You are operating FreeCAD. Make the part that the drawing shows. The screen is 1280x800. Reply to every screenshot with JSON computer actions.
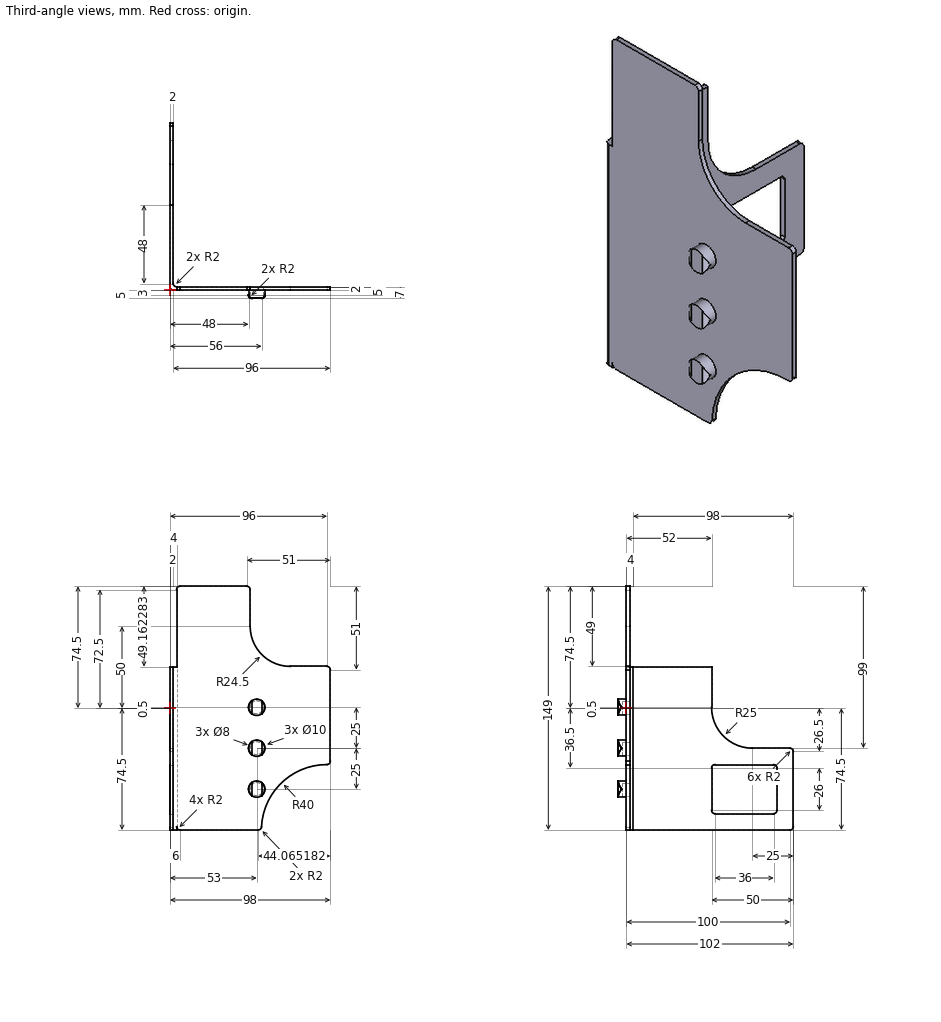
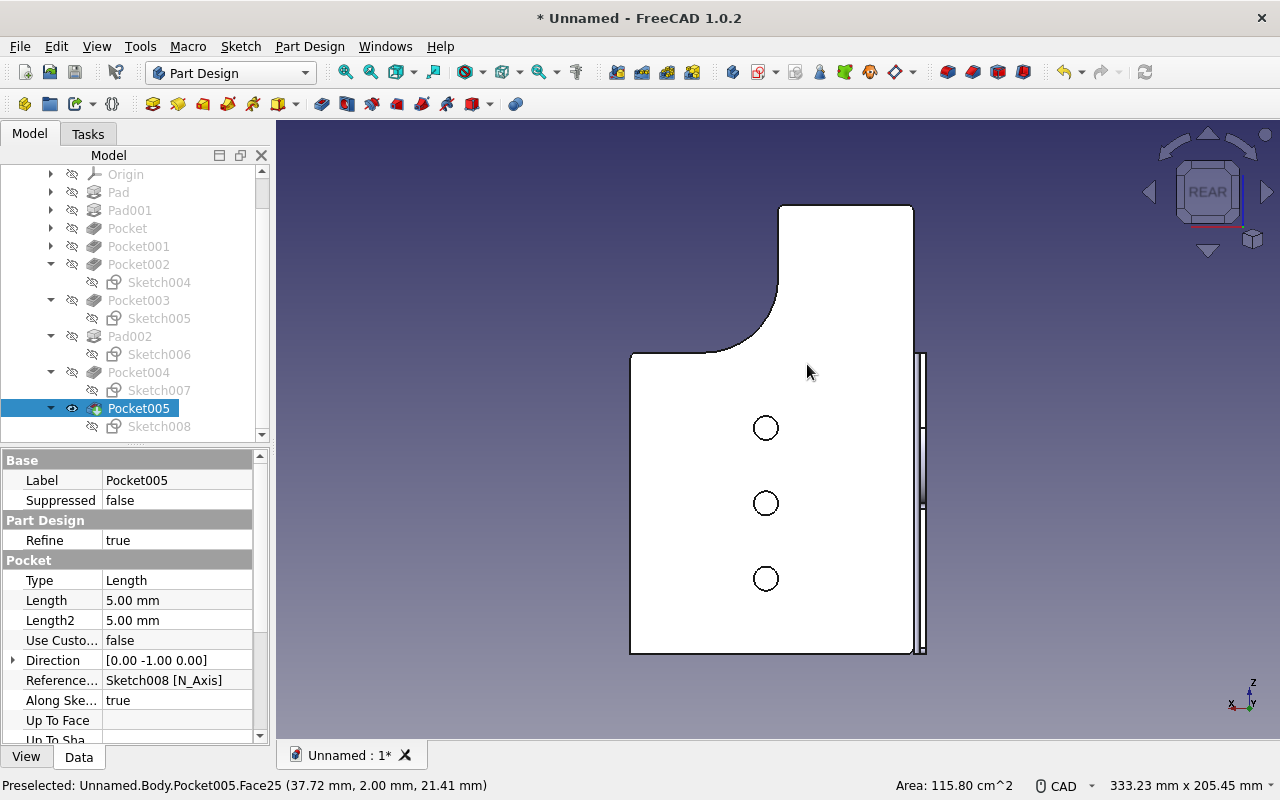
{"action": "left_click", "coordinate": [758, 72]}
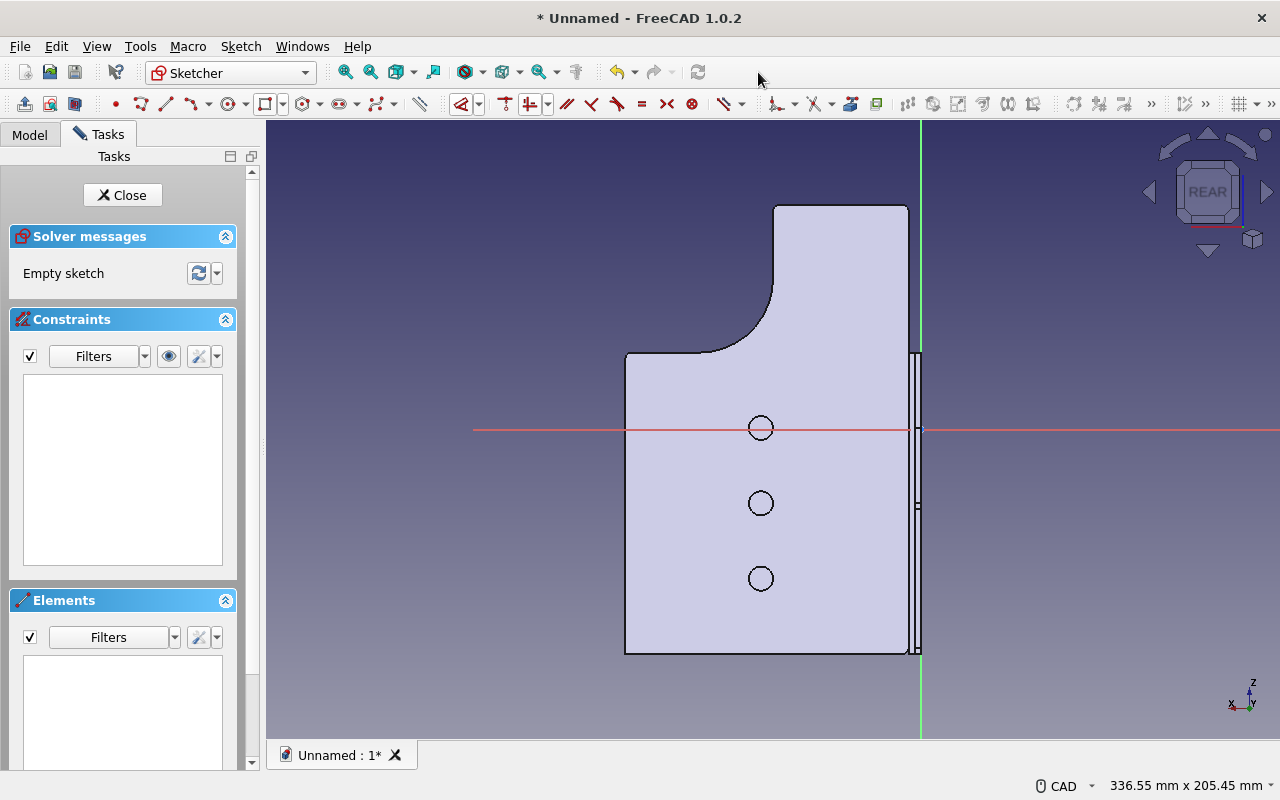
{"action": "scroll", "coordinate": [856, 678], "scroll_direction": "up", "scroll_amount": 3}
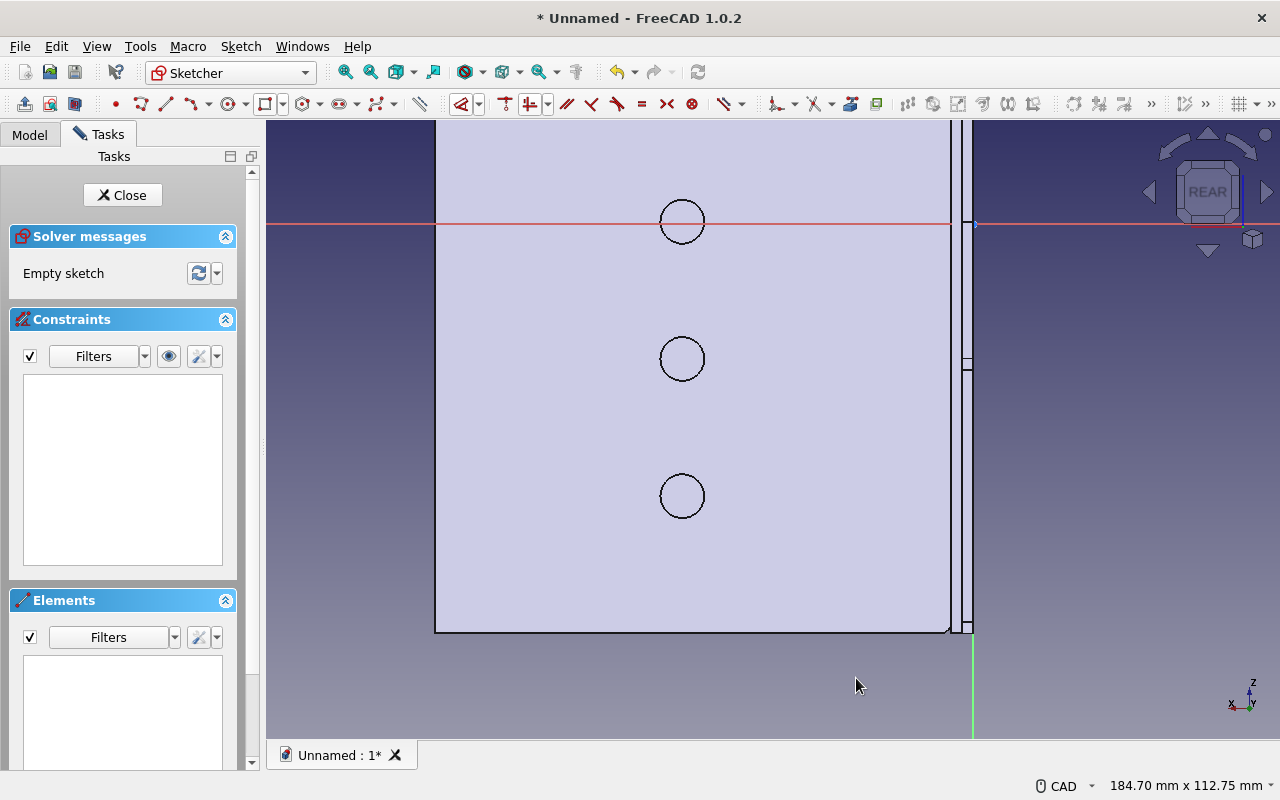
{"action": "key", "text": "g m"}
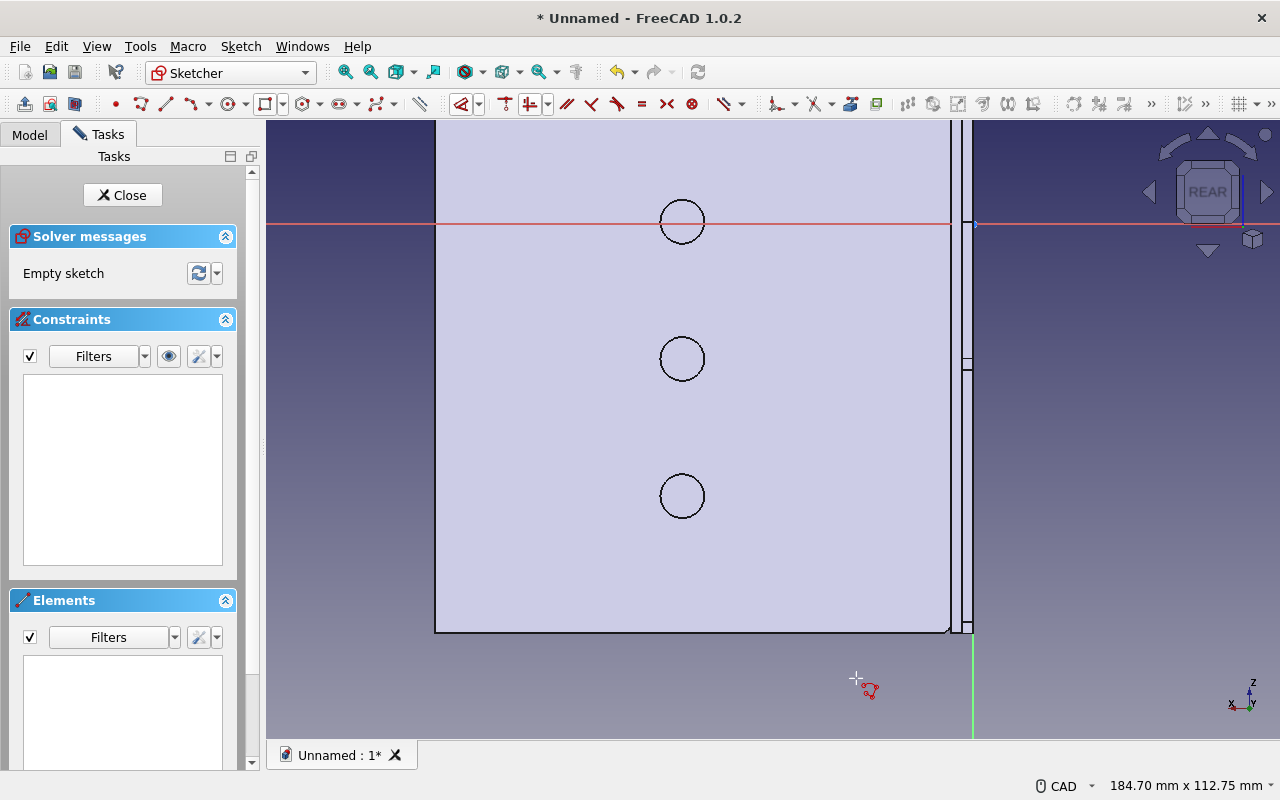
{"action": "left_click", "coordinate": [435, 403]}
{"action": "left_click", "coordinate": [435, 633]}
{"action": "left_click", "coordinate": [677, 633]}
{"action": "right_click", "coordinate": [677, 633]}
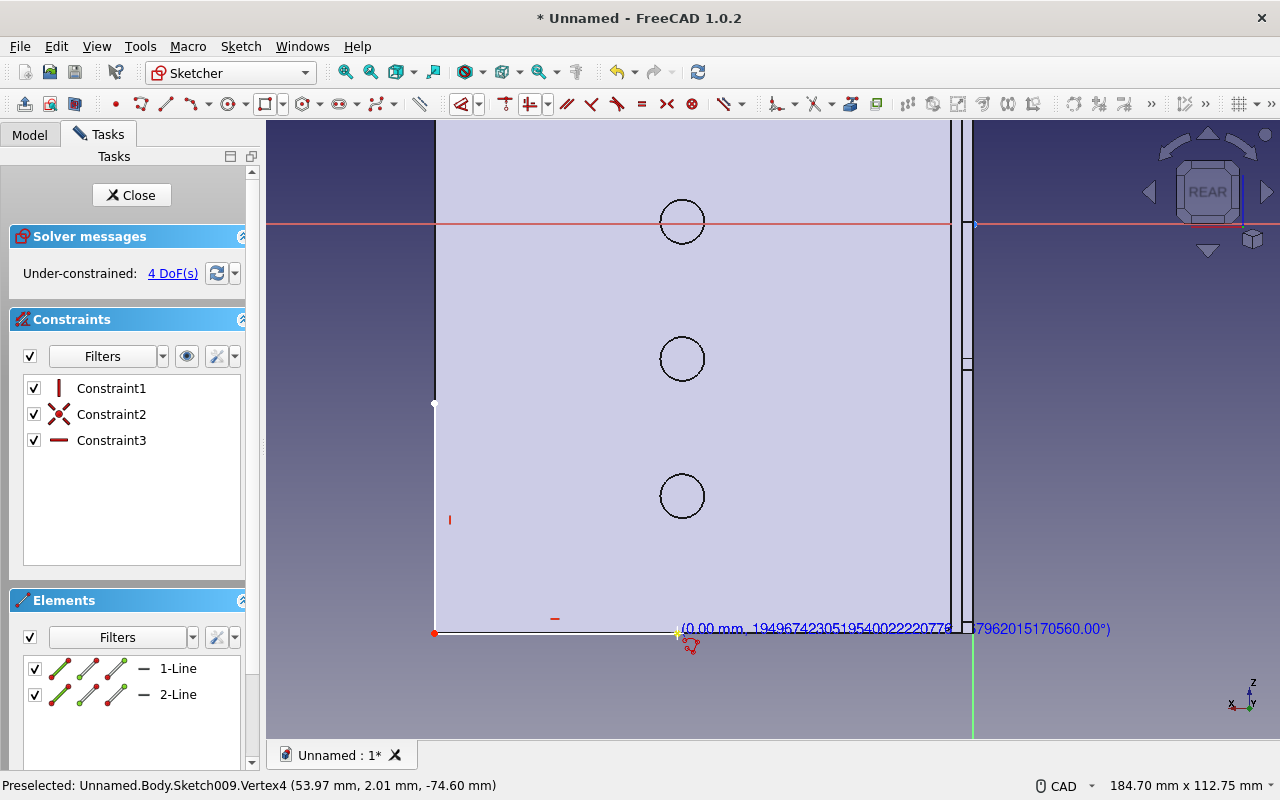
{"action": "key", "text": "g 3 a"}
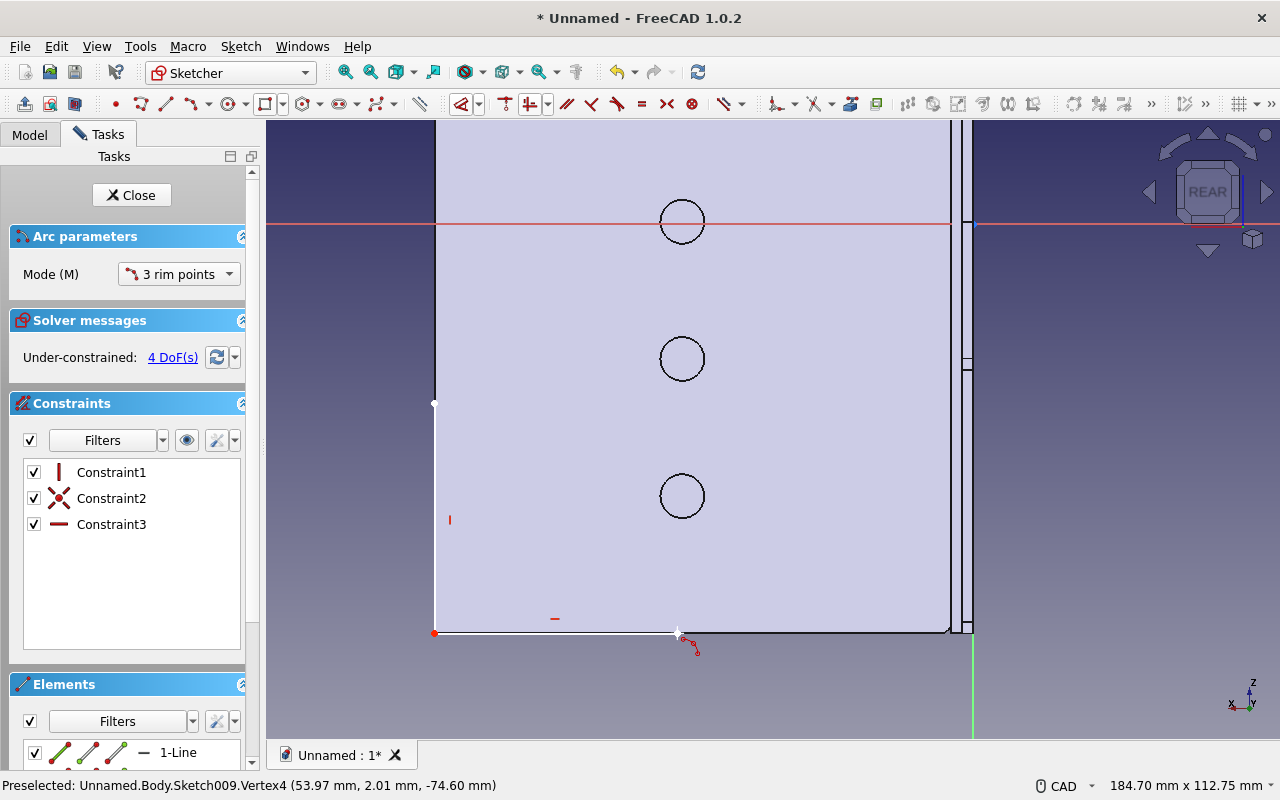
{"action": "left_click", "coordinate": [677, 634]}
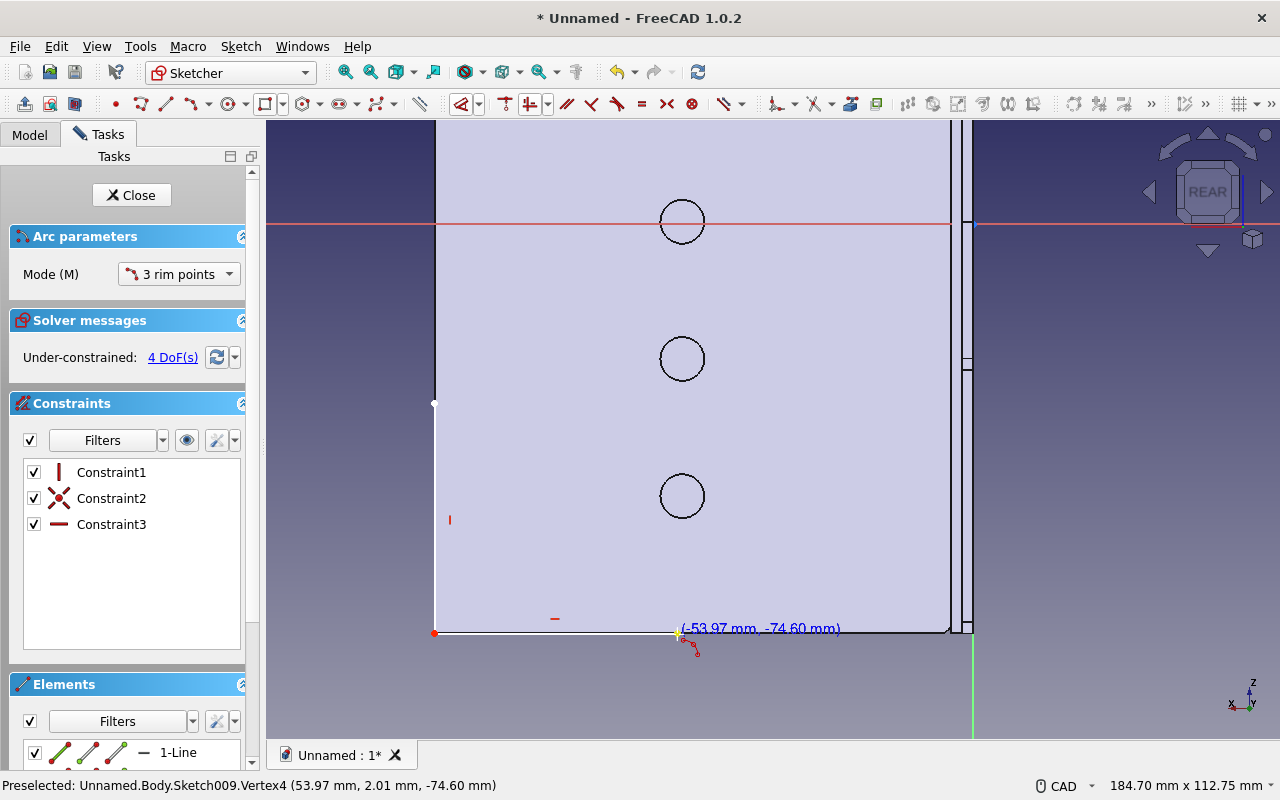
{"action": "scroll", "coordinate": [666, 623], "scroll_direction": "up", "scroll_amount": 3}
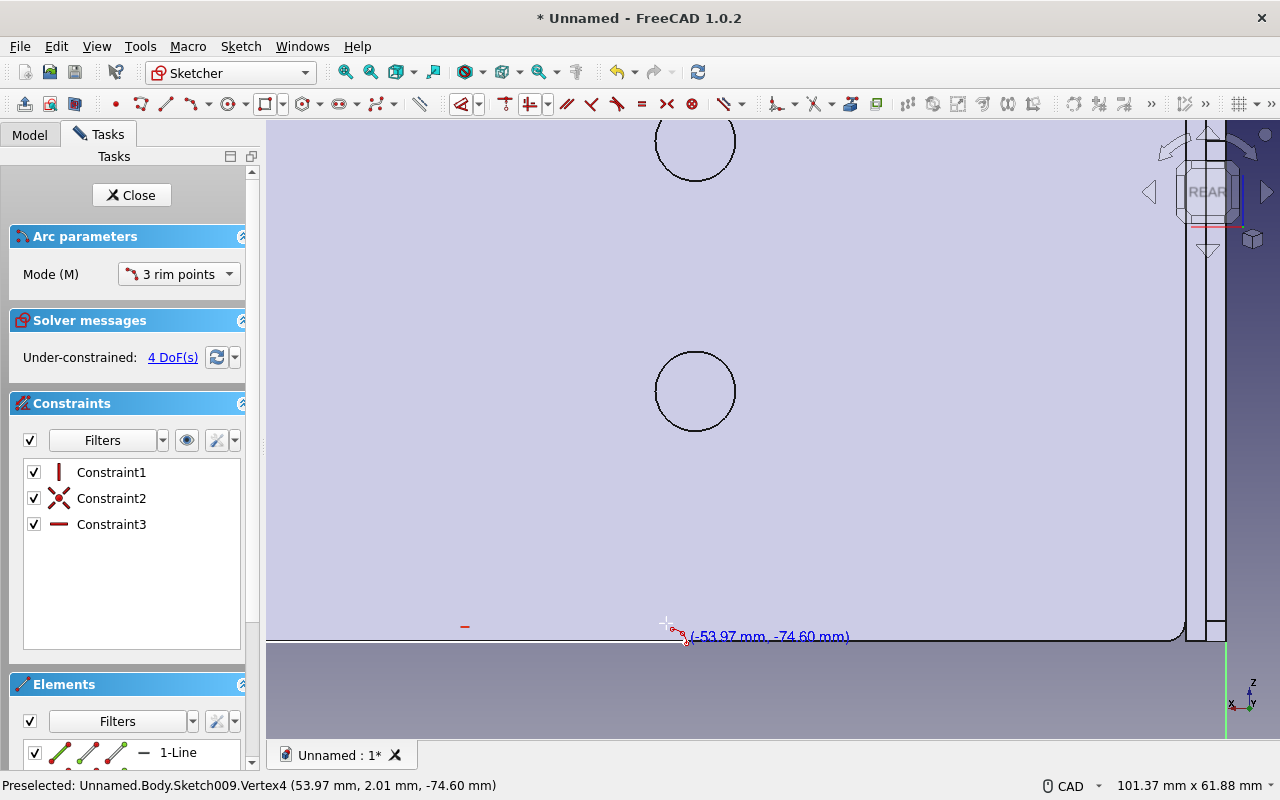
{"action": "left_click", "coordinate": [666, 622]}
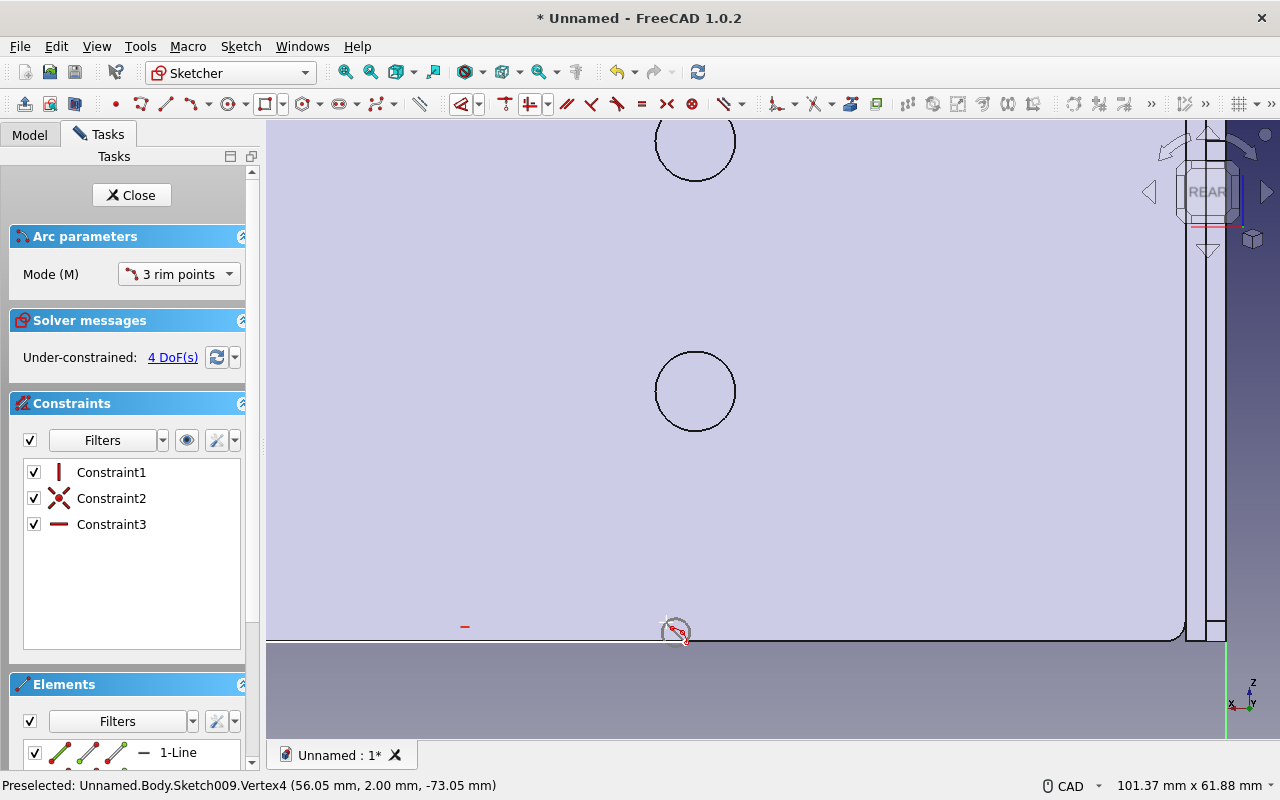
{"action": "scroll", "coordinate": [672, 636], "scroll_direction": "up", "scroll_amount": 6}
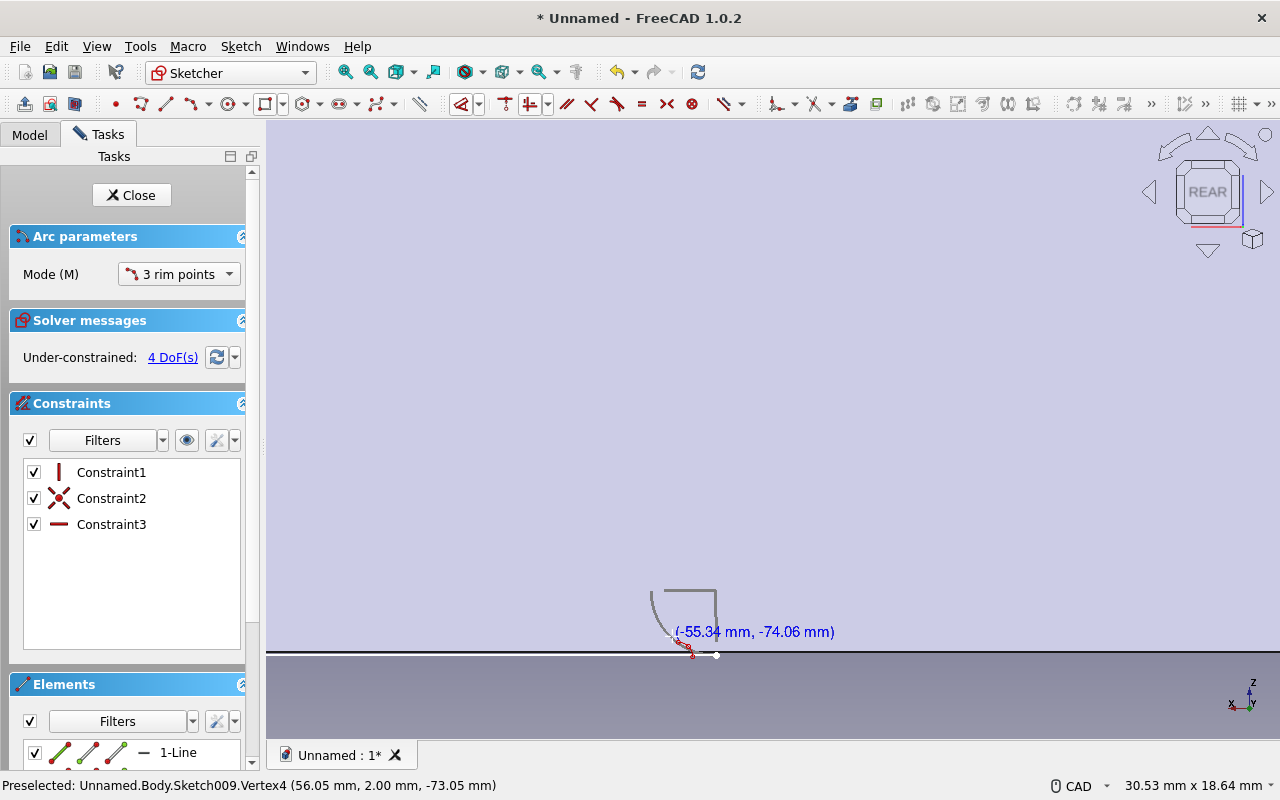
{"action": "left_click", "coordinate": [672, 634]}